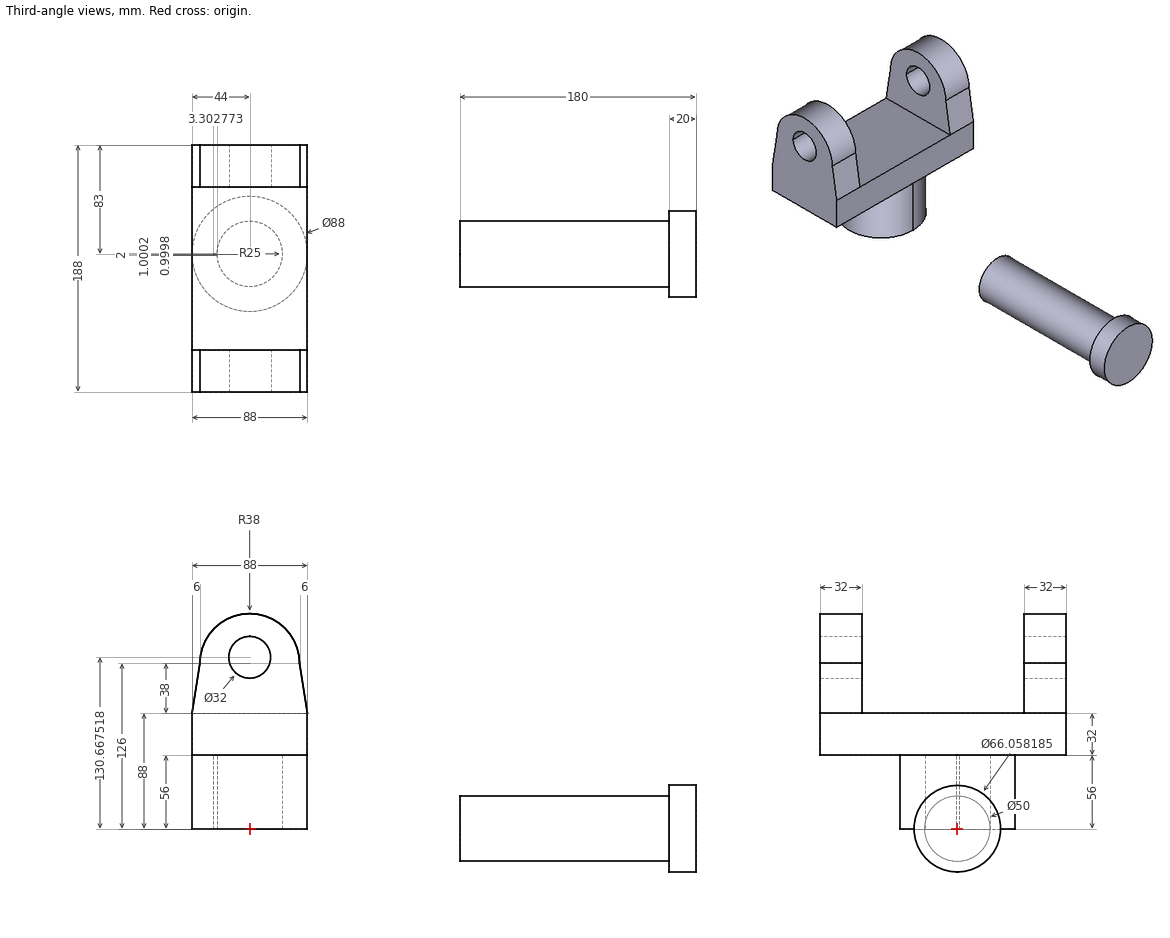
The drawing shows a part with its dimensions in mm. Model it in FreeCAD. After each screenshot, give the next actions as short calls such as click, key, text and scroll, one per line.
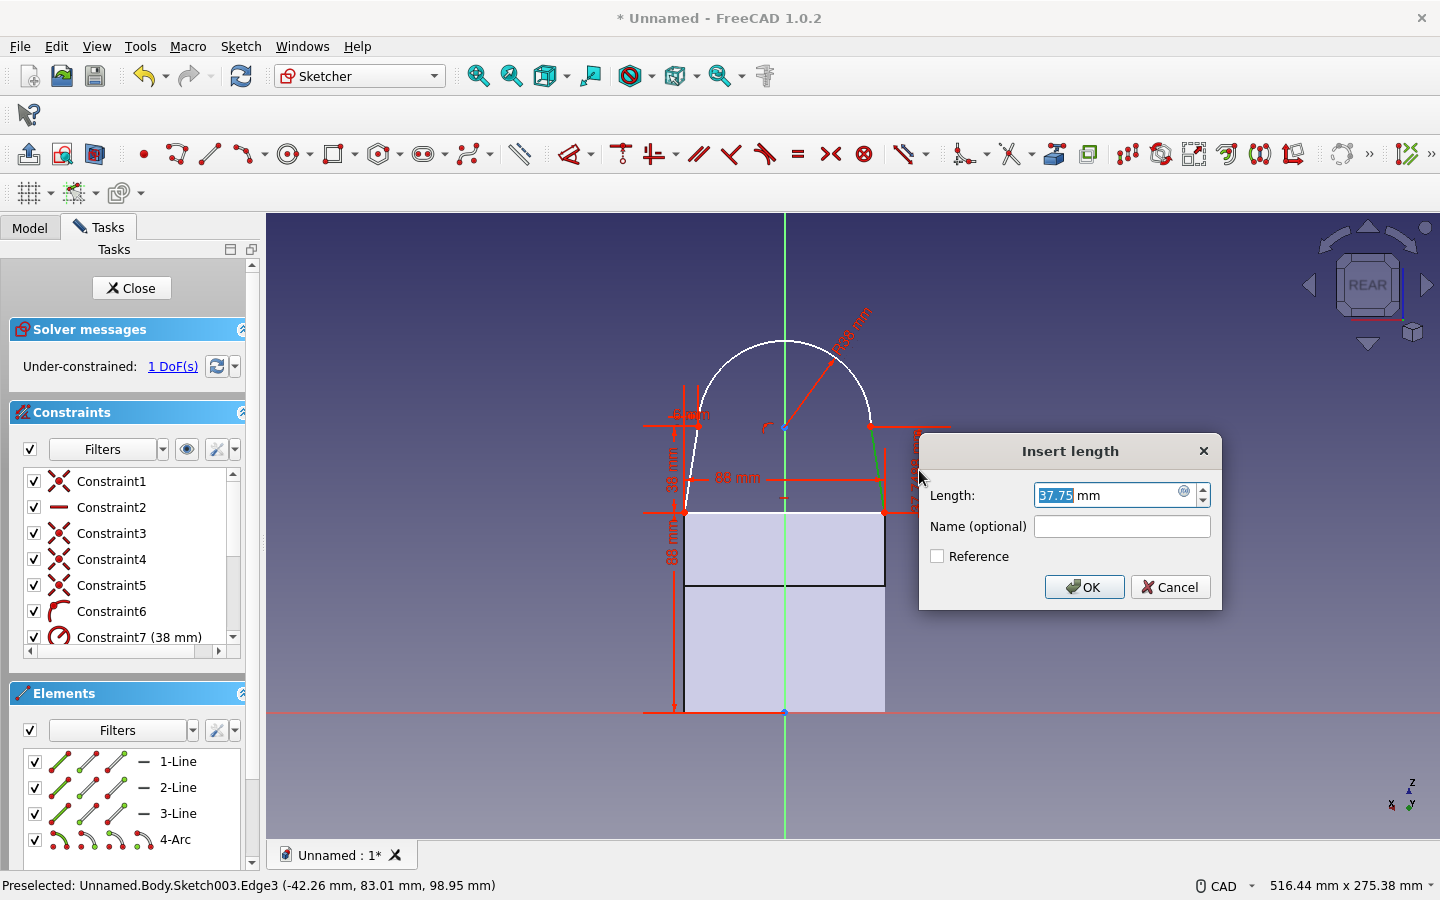
text(38)
key(Return)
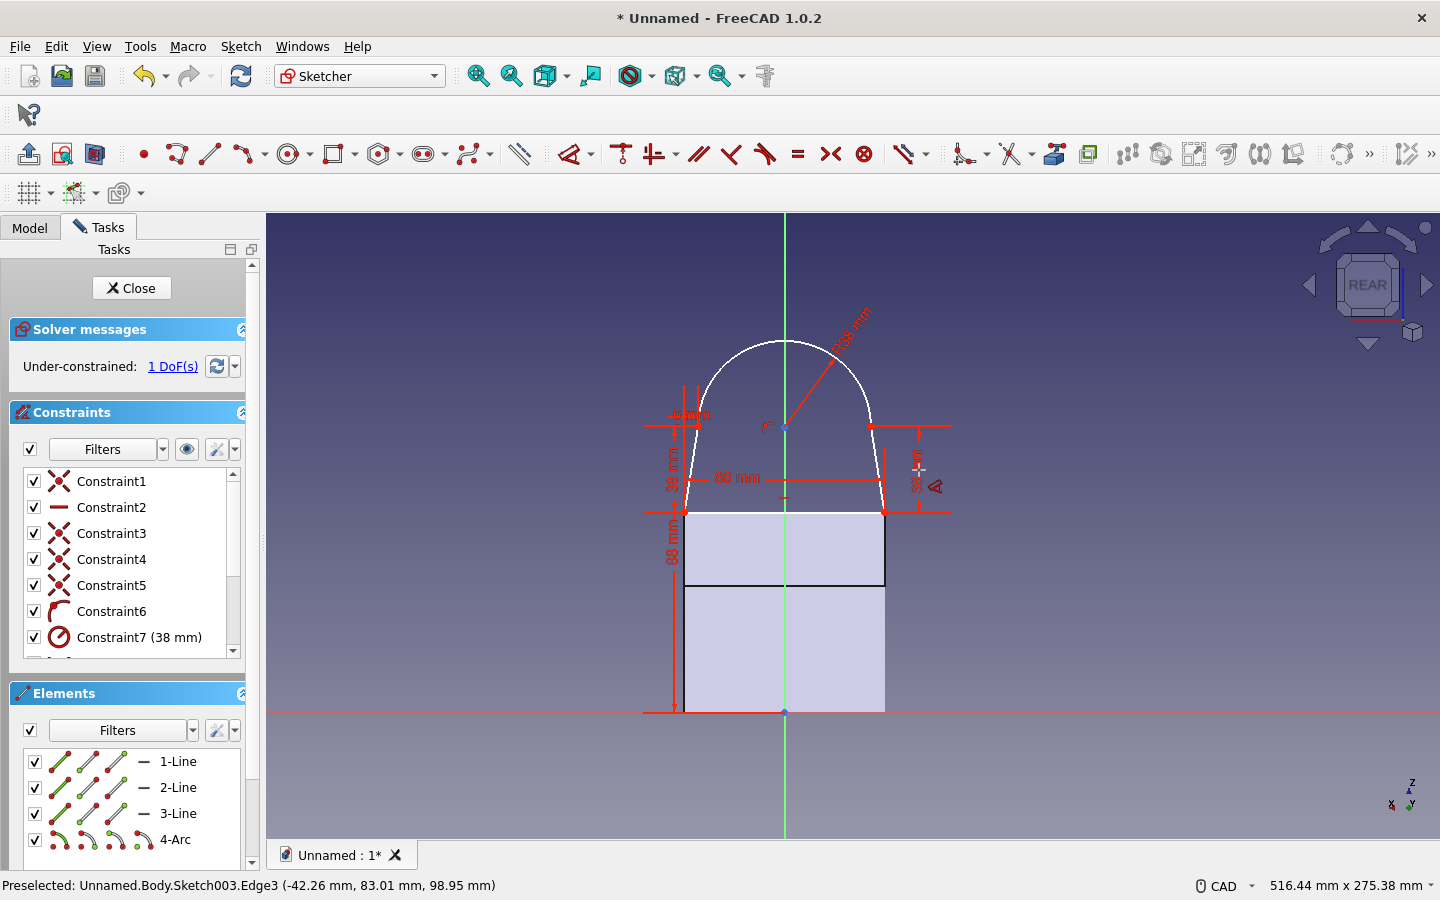
click(785, 427)
click(819, 570)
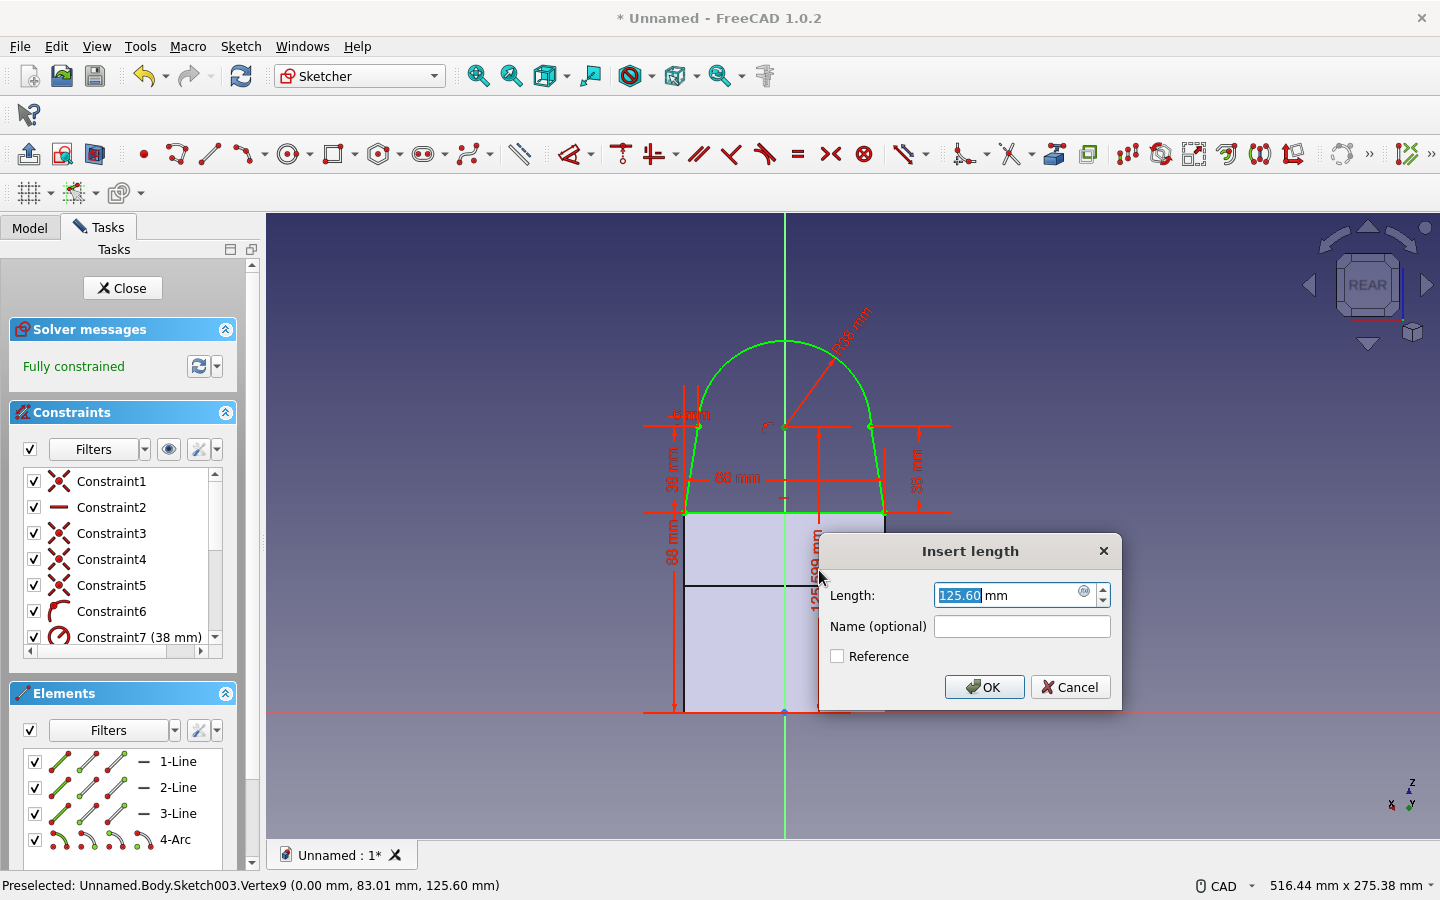
text(126)
key(Return)
key(Escape)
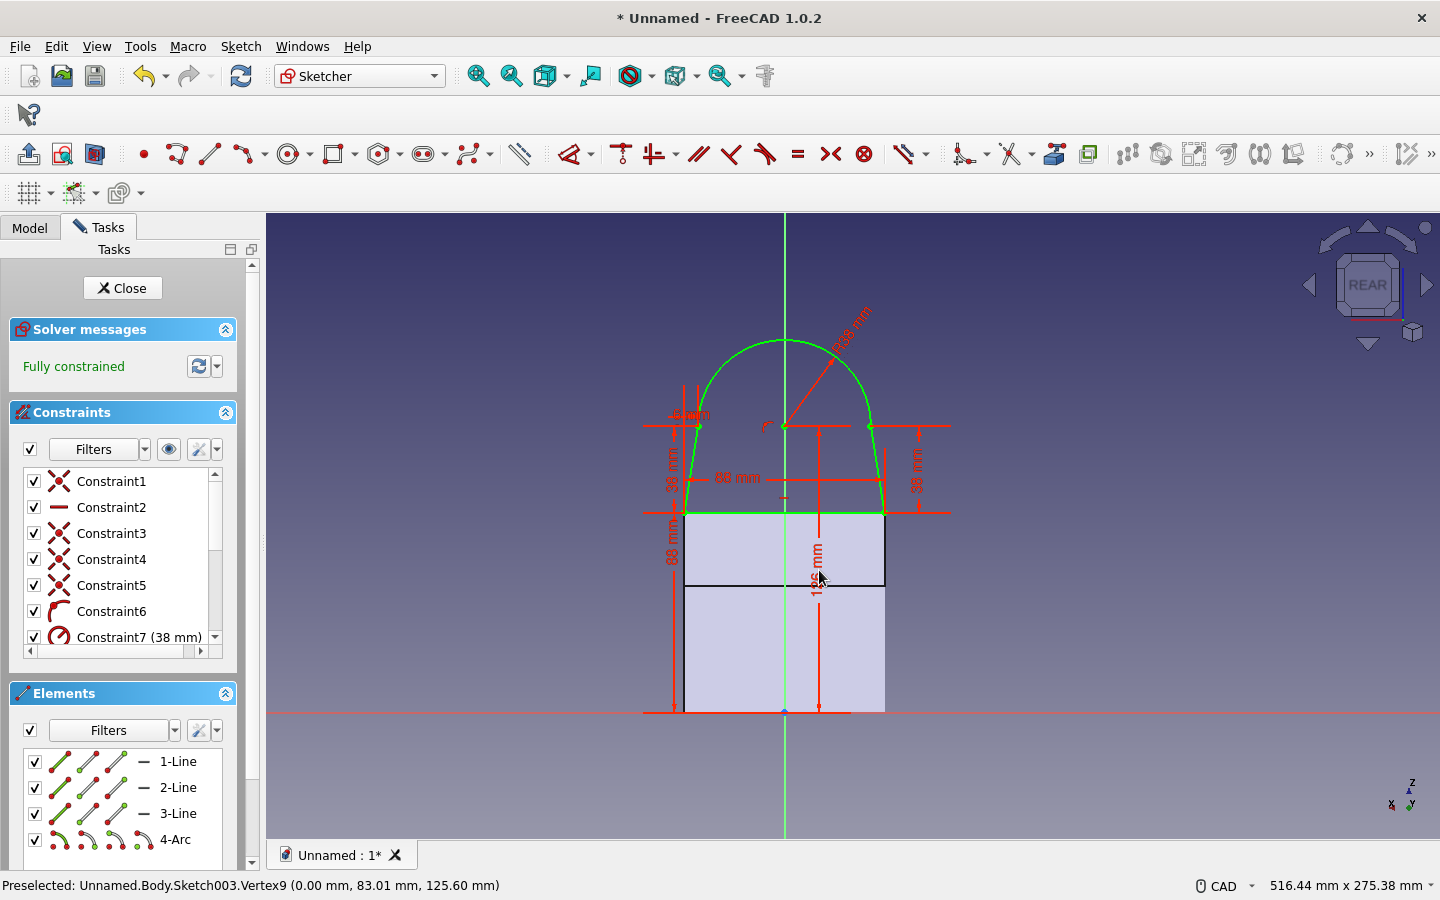
click(123, 288)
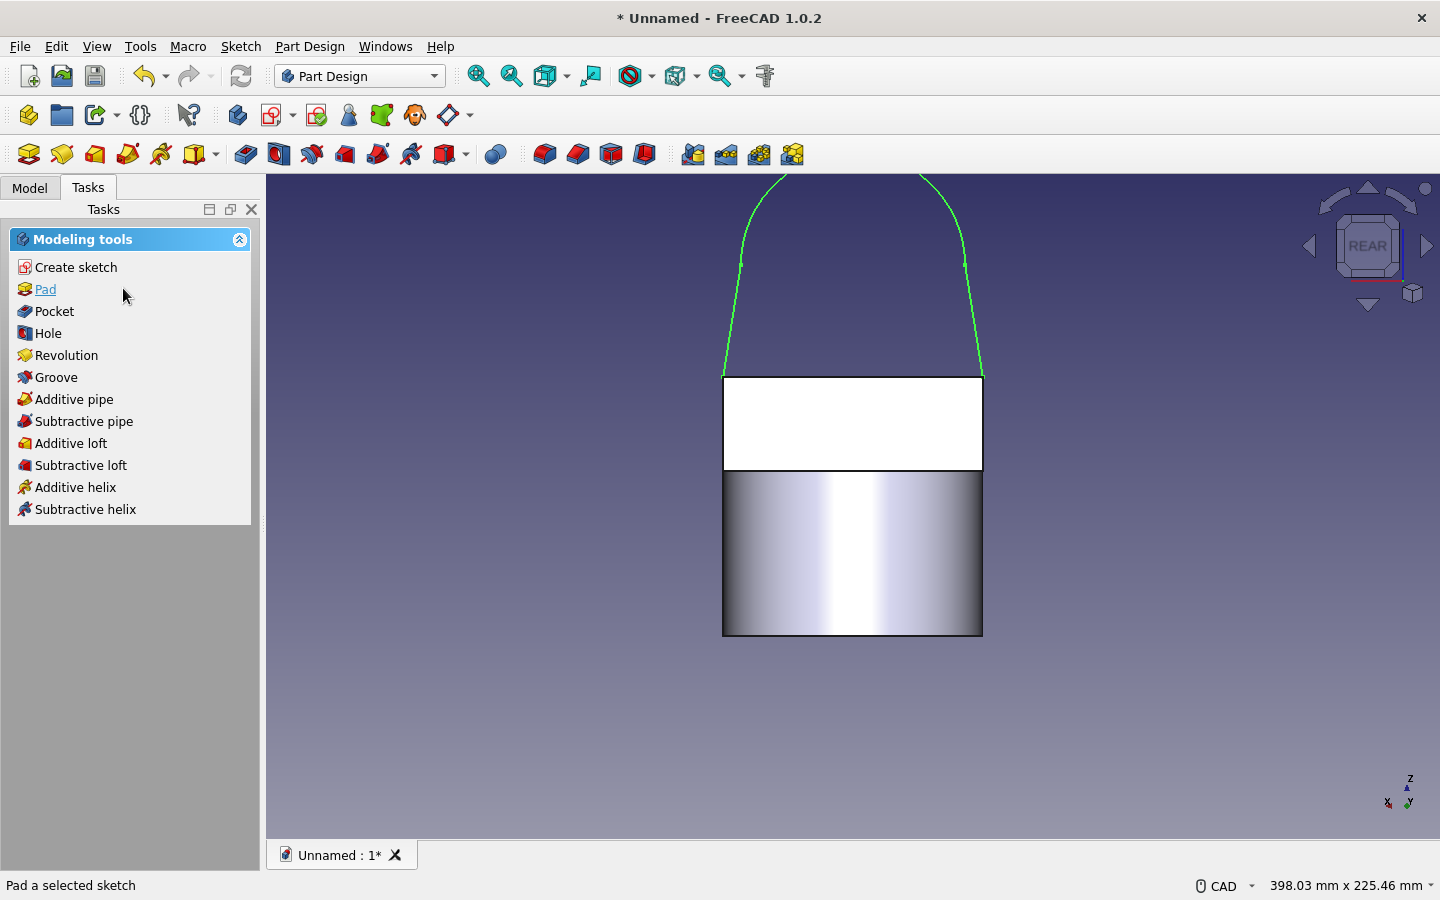
click(29, 154)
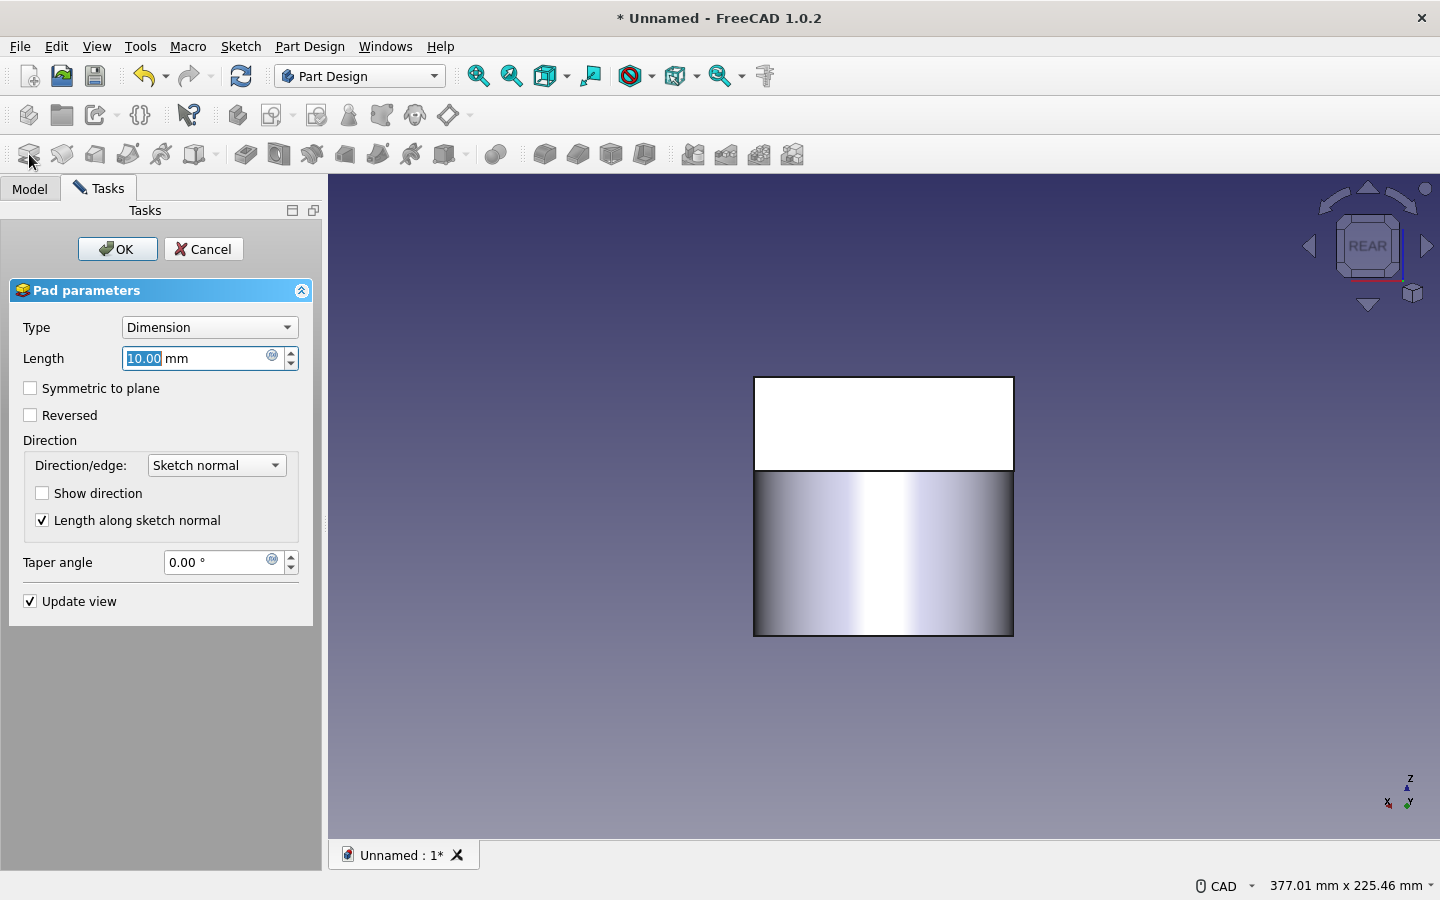
text(32)
key(Tab)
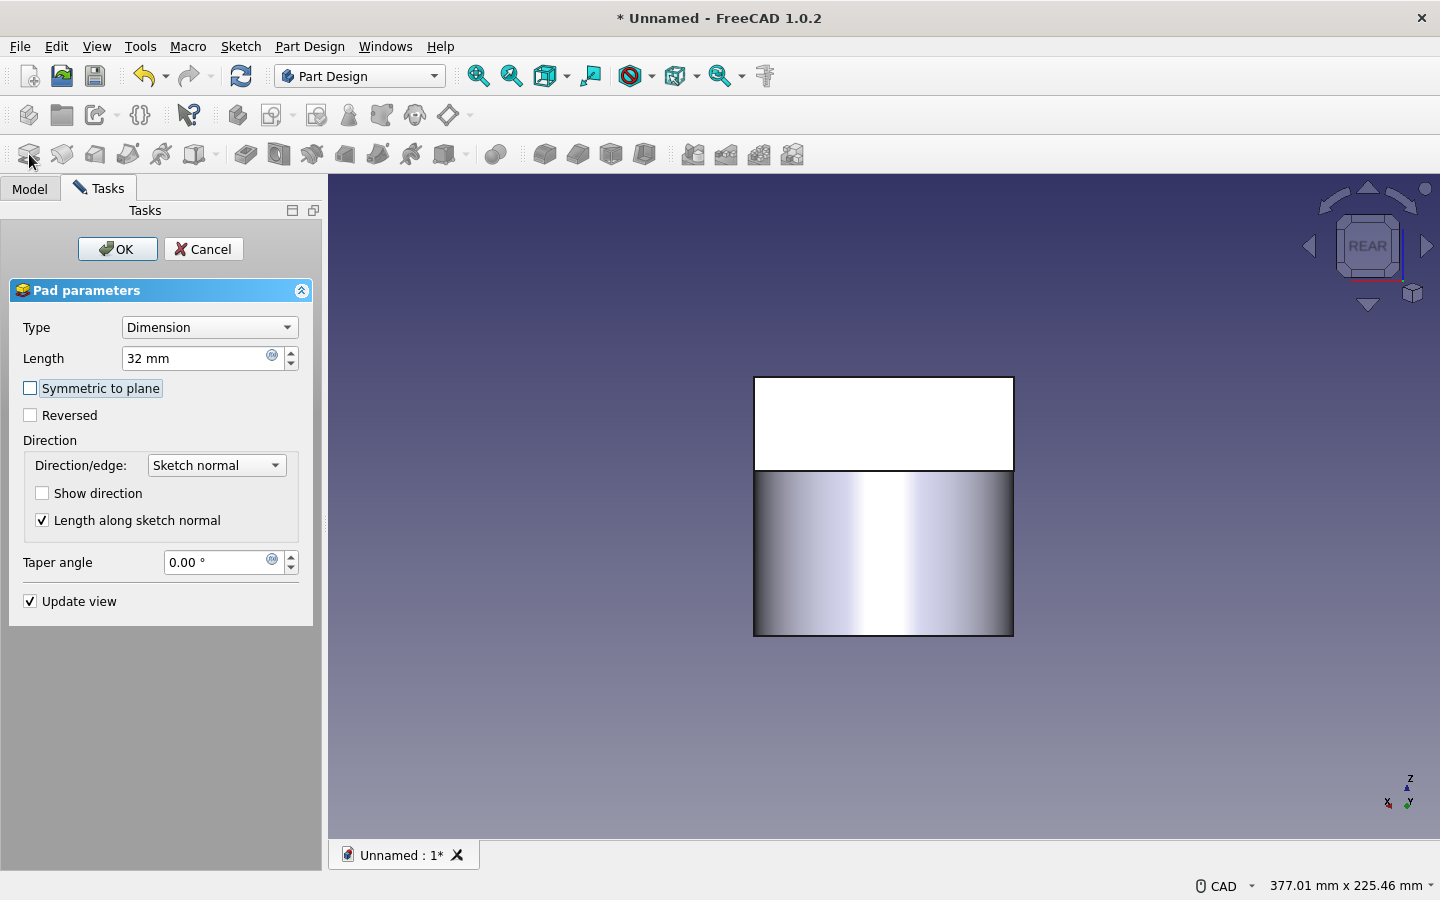
click(31, 415)